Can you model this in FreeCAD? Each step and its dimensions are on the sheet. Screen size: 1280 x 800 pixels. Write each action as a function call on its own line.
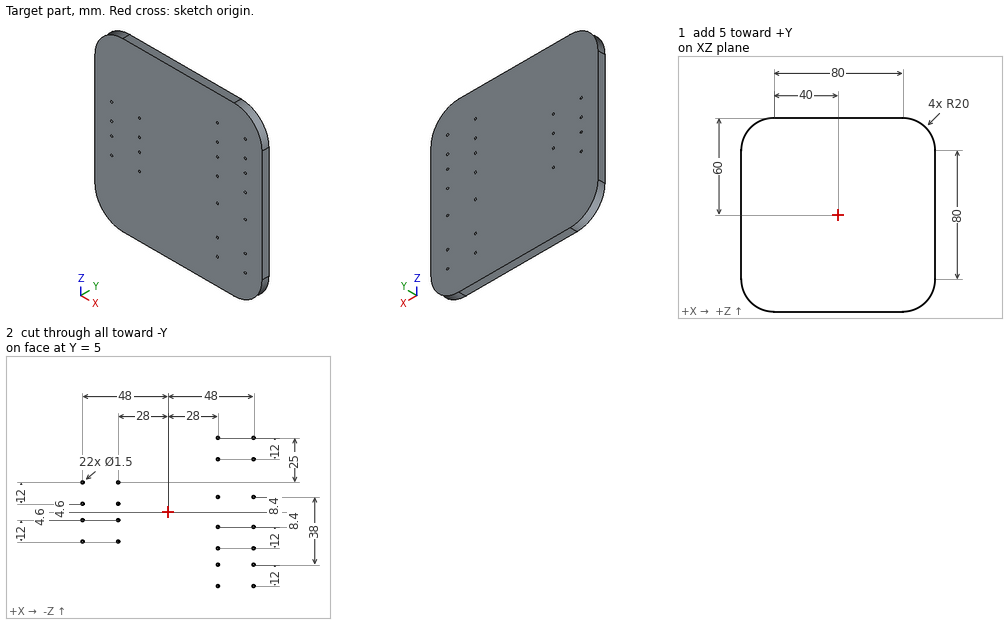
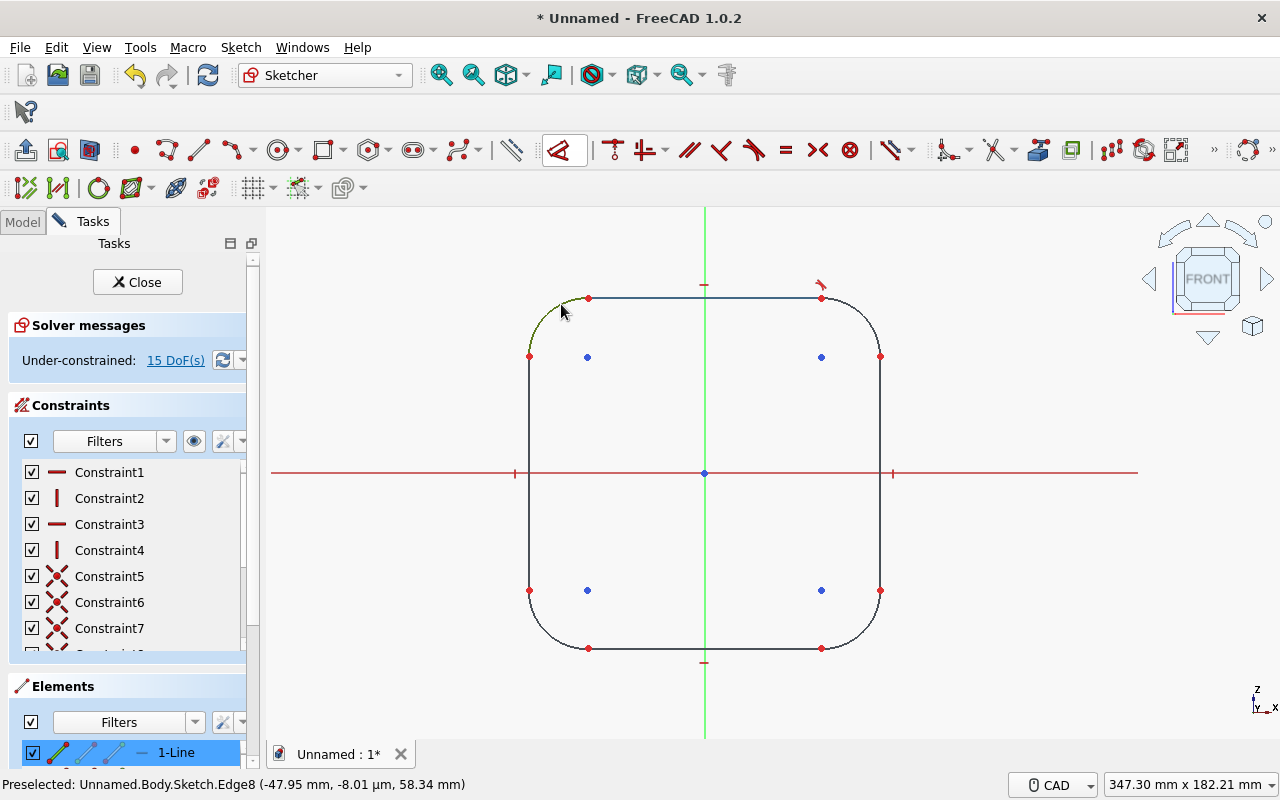
click(754, 150)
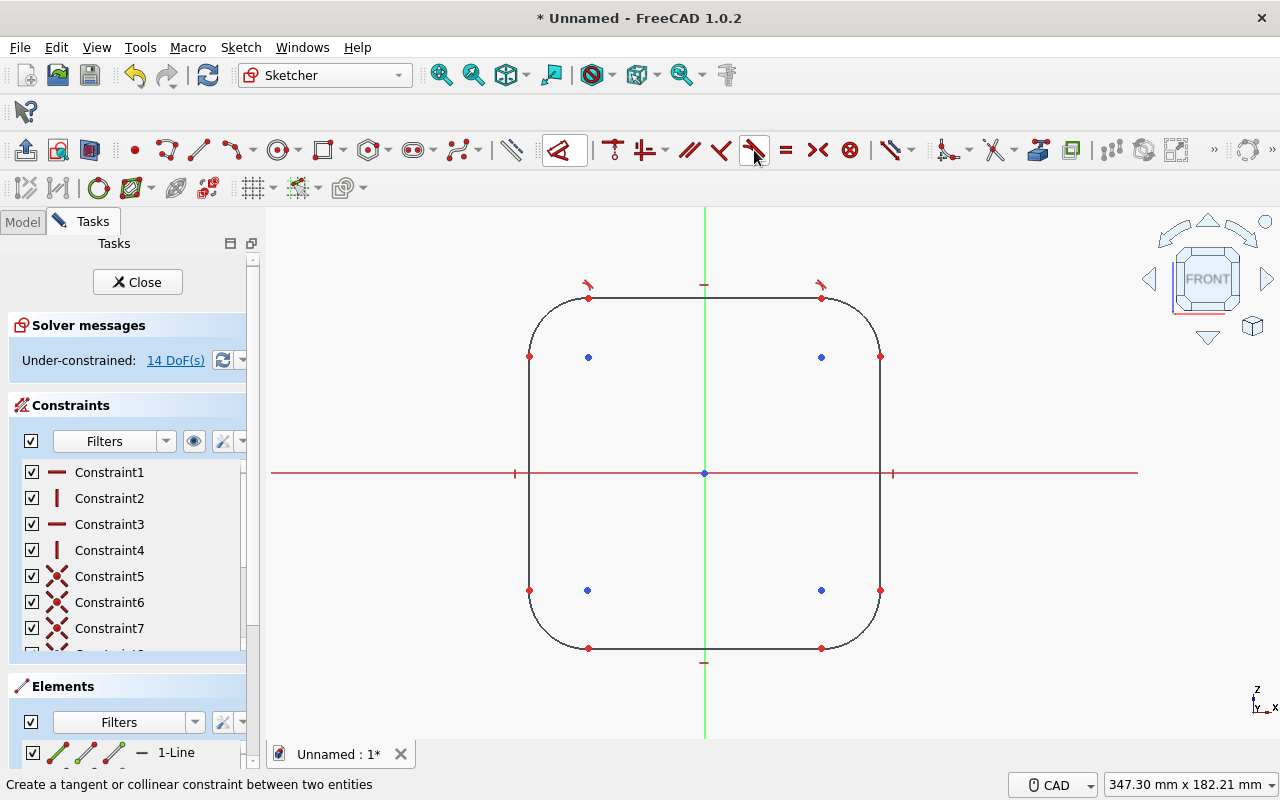
click(880, 427)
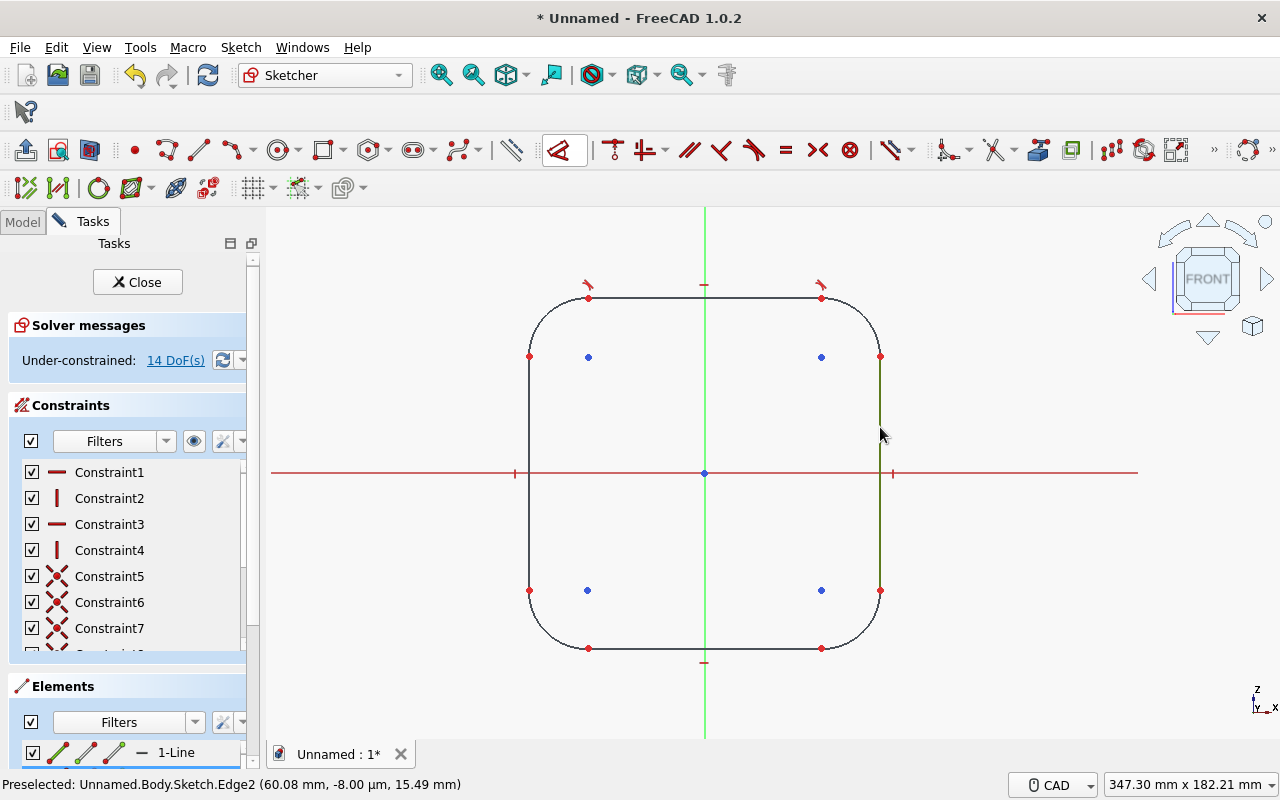
click(874, 330)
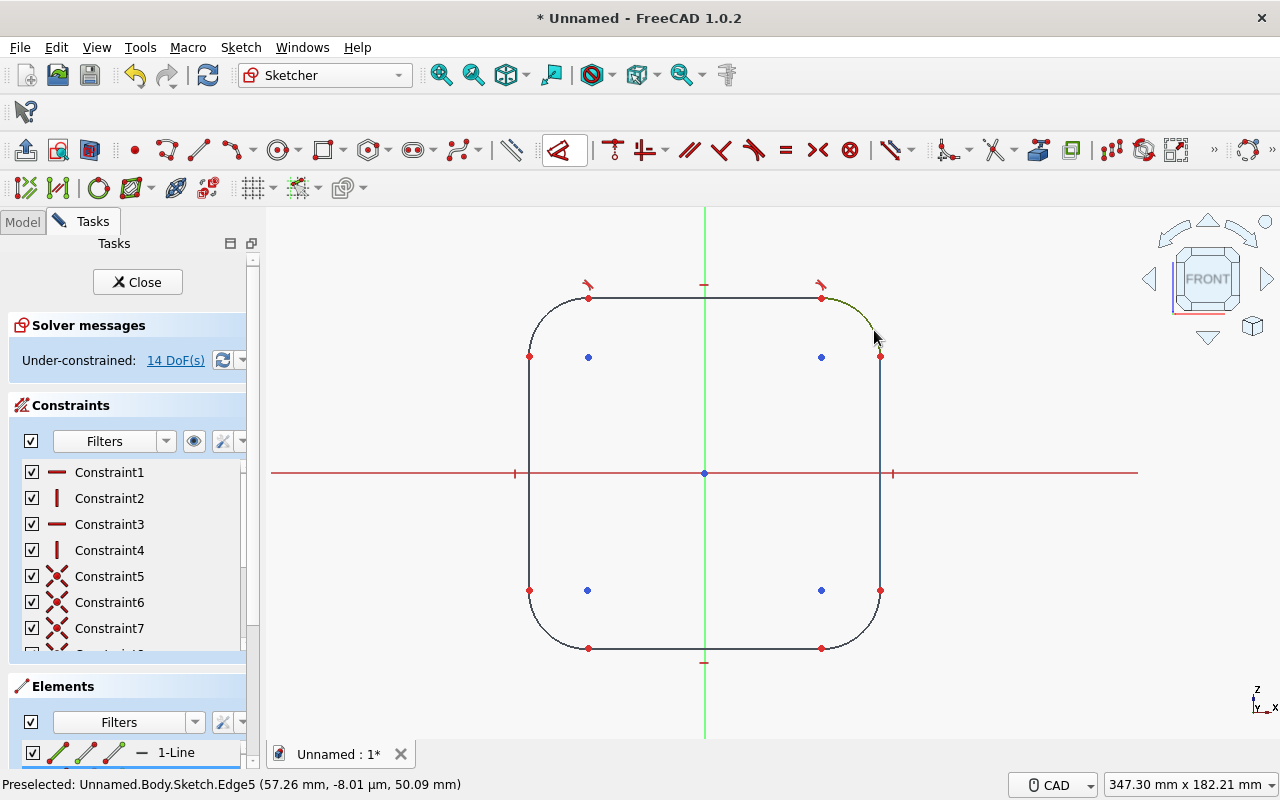
click(754, 150)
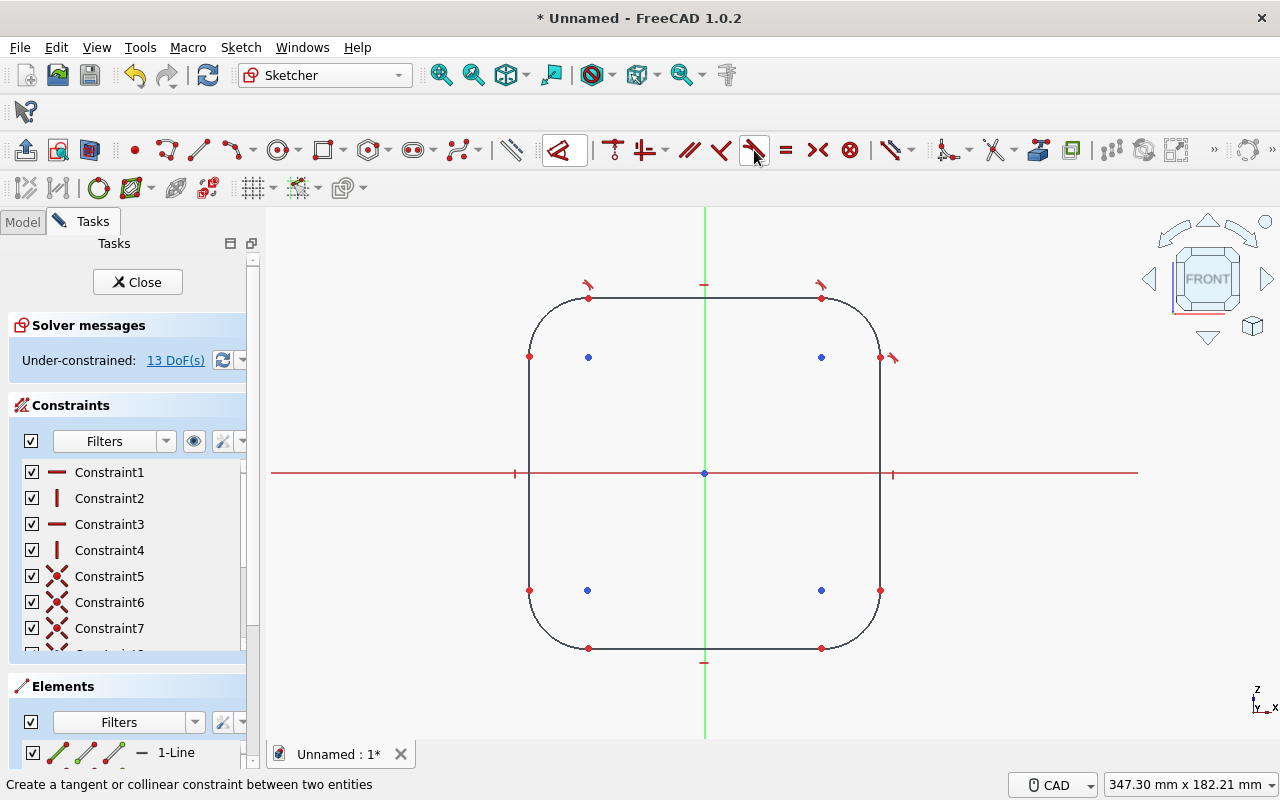
click(880, 427)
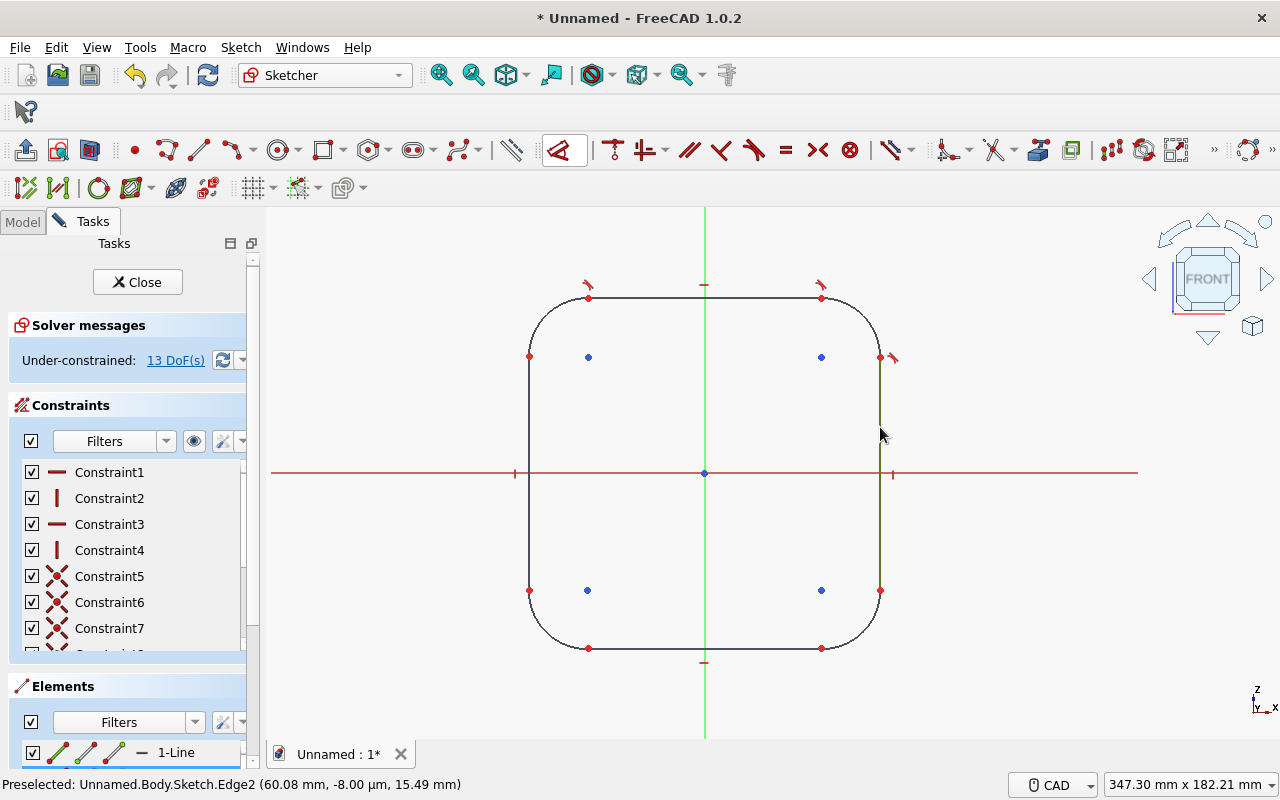
click(848, 643)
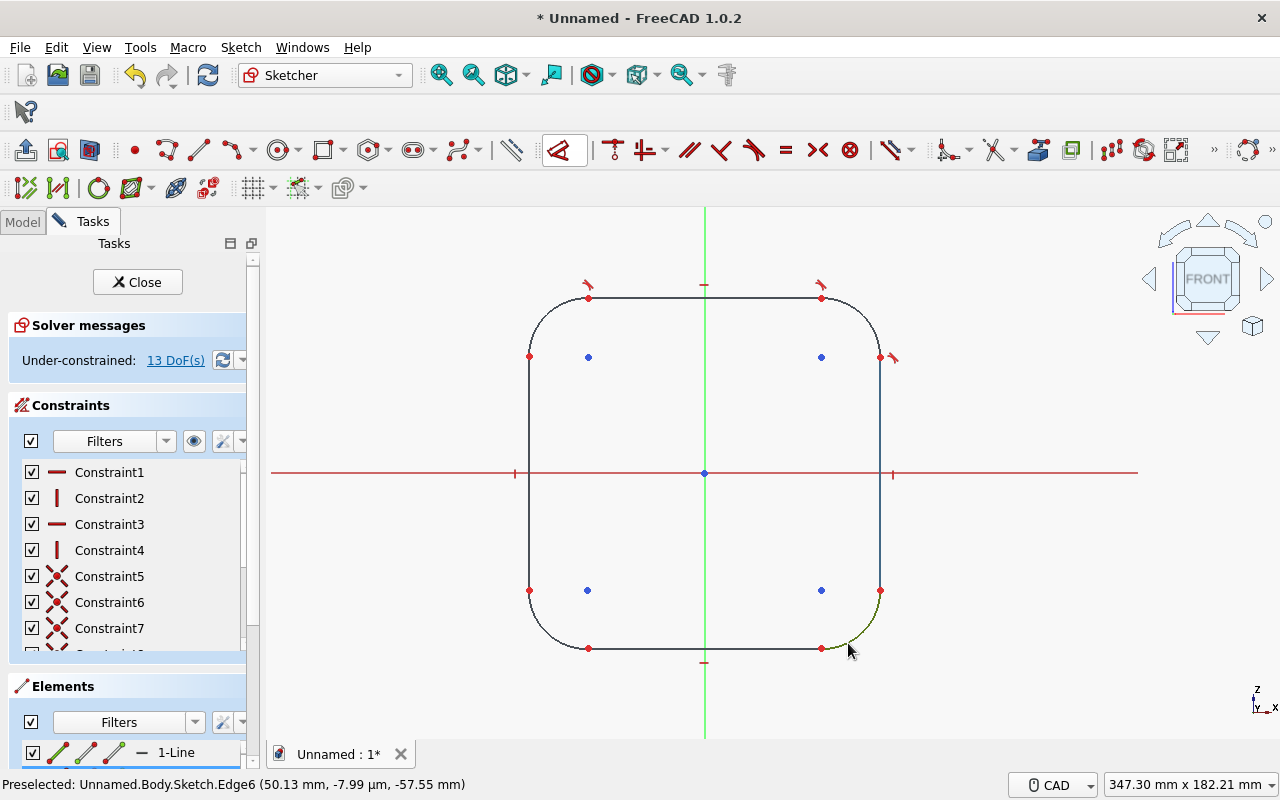
click(754, 150)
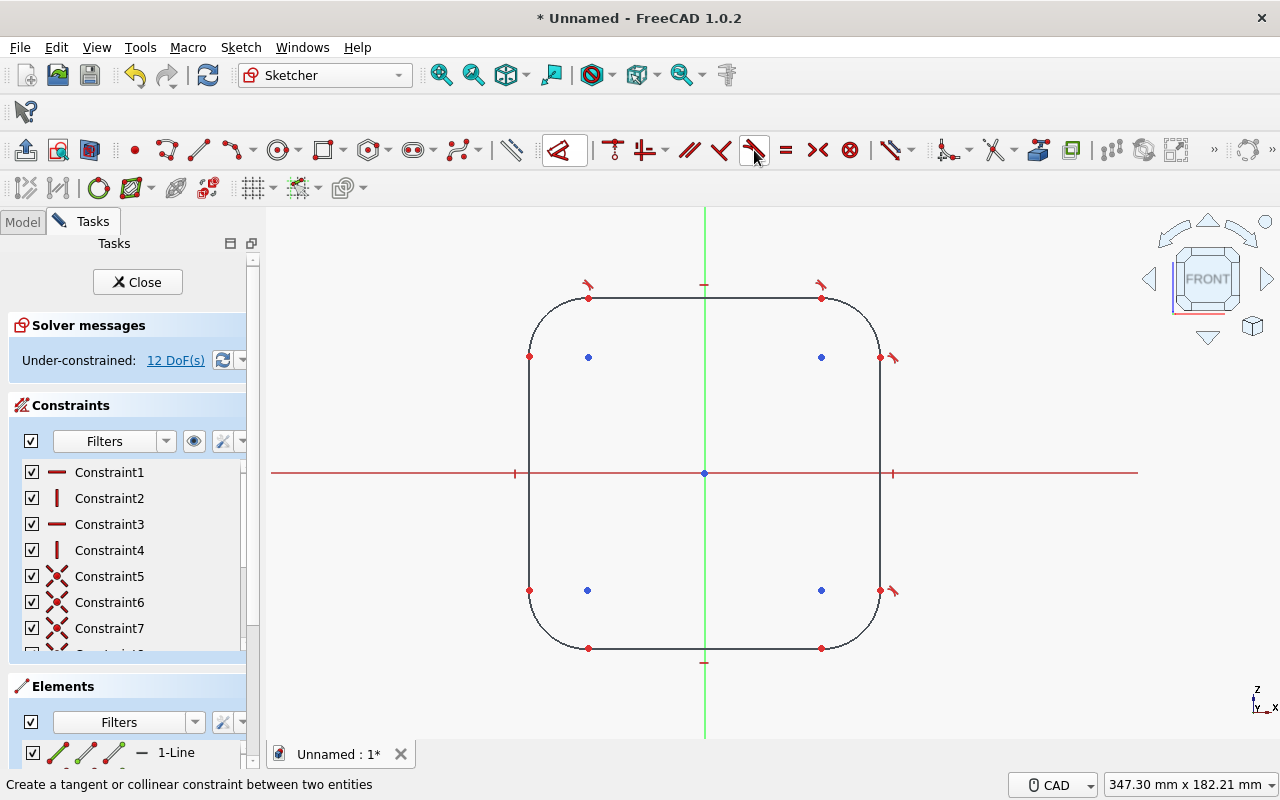
click(751, 649)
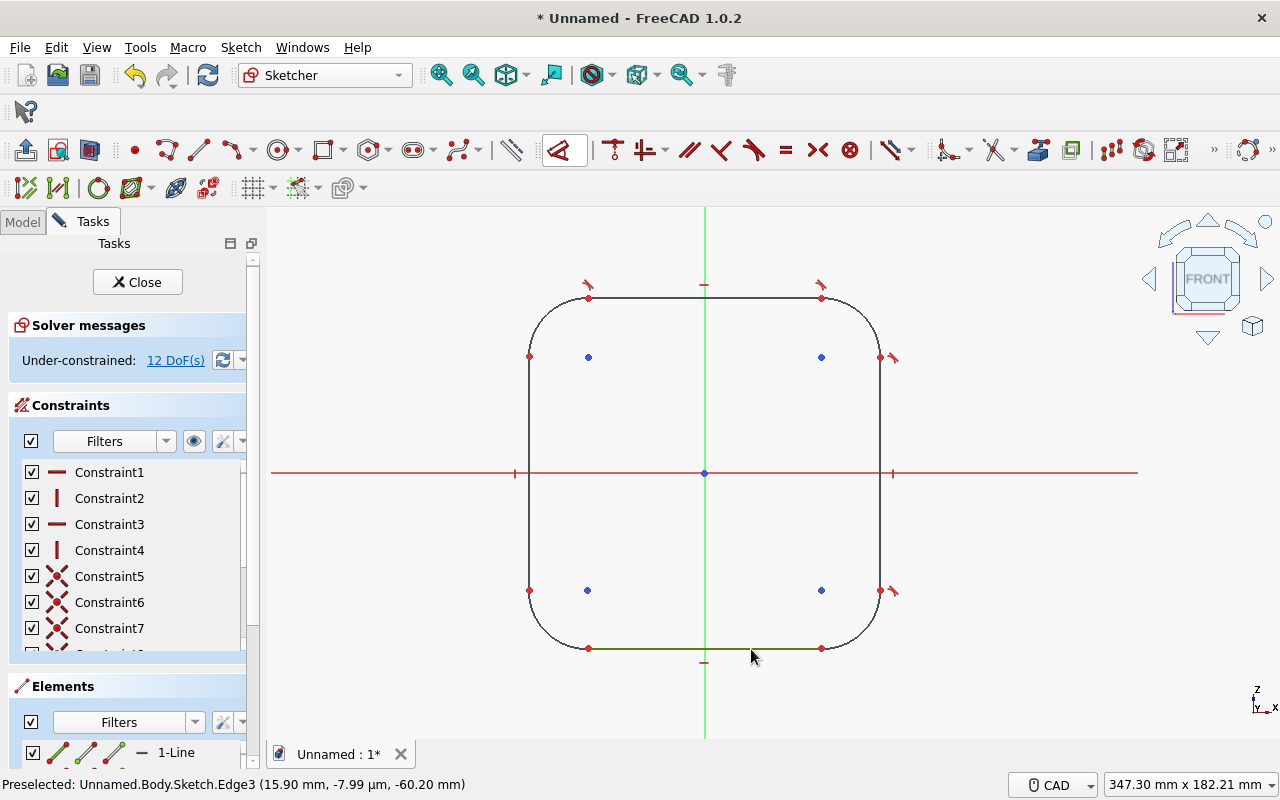
click(848, 643)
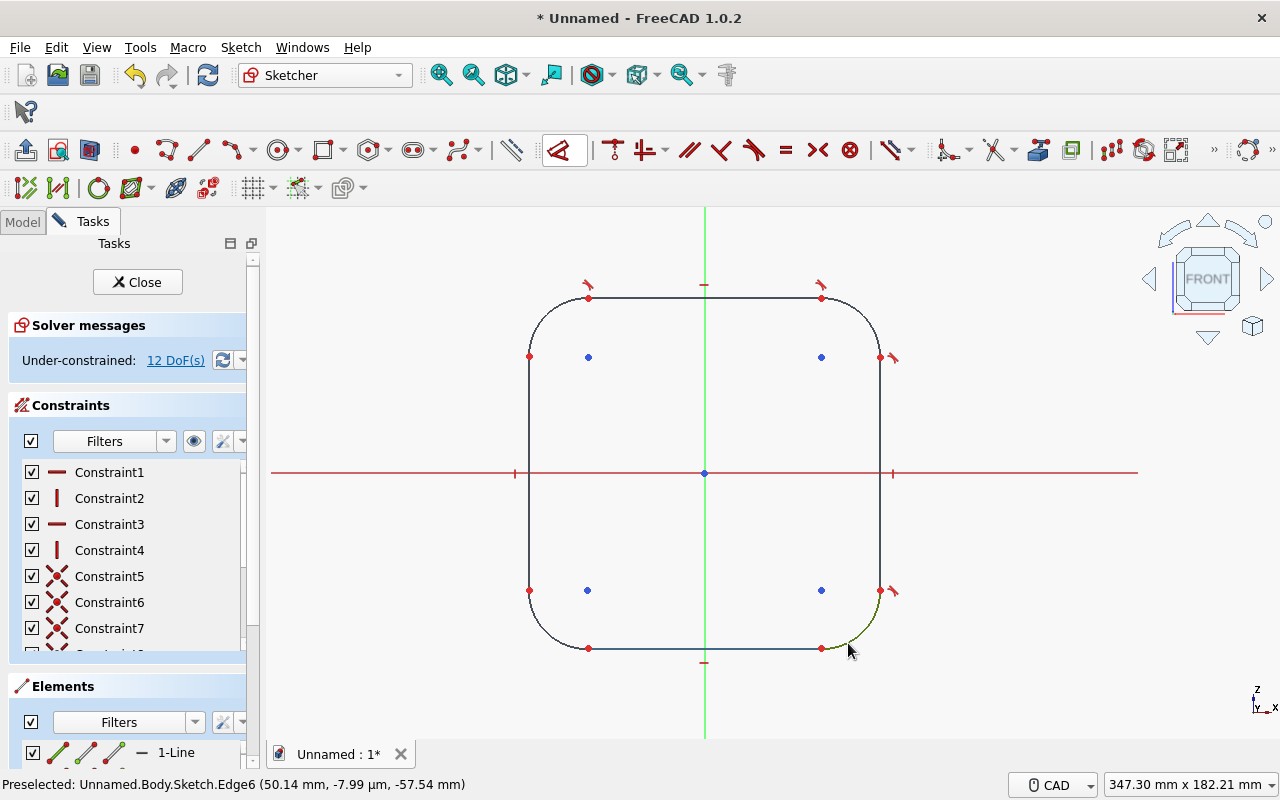
click(754, 150)